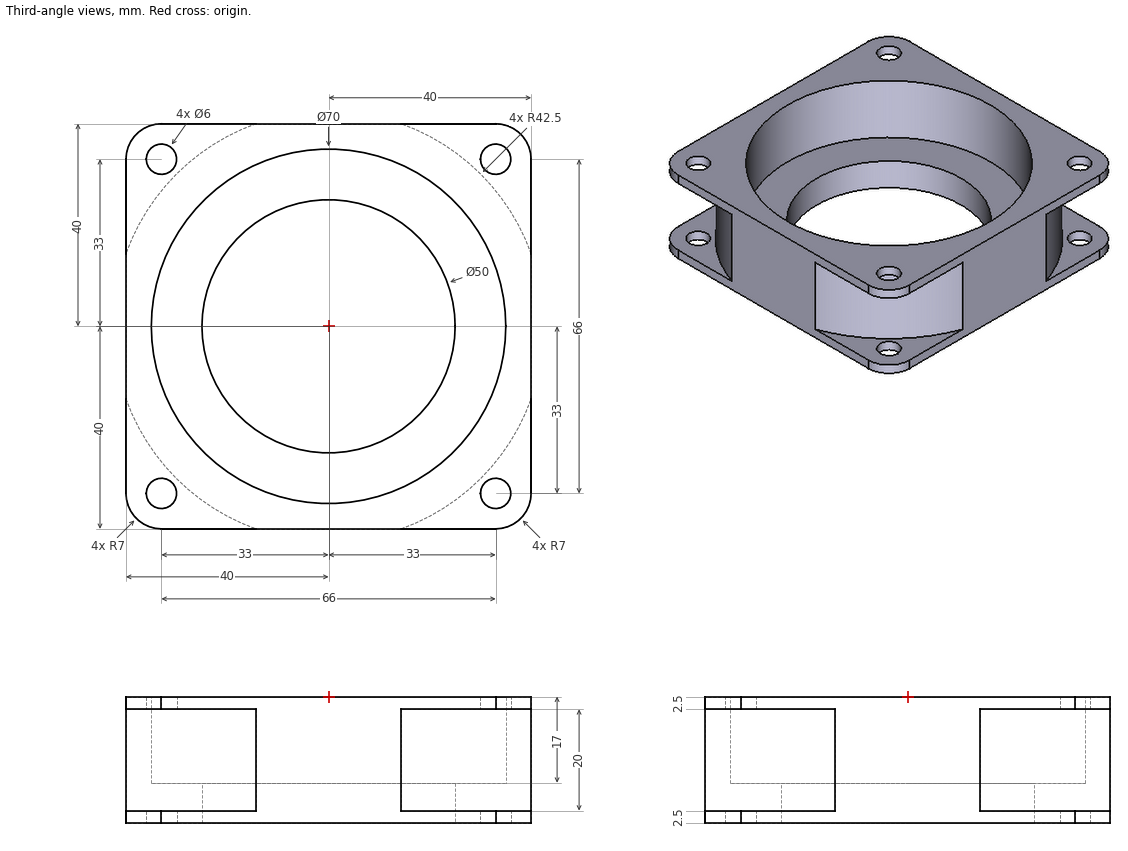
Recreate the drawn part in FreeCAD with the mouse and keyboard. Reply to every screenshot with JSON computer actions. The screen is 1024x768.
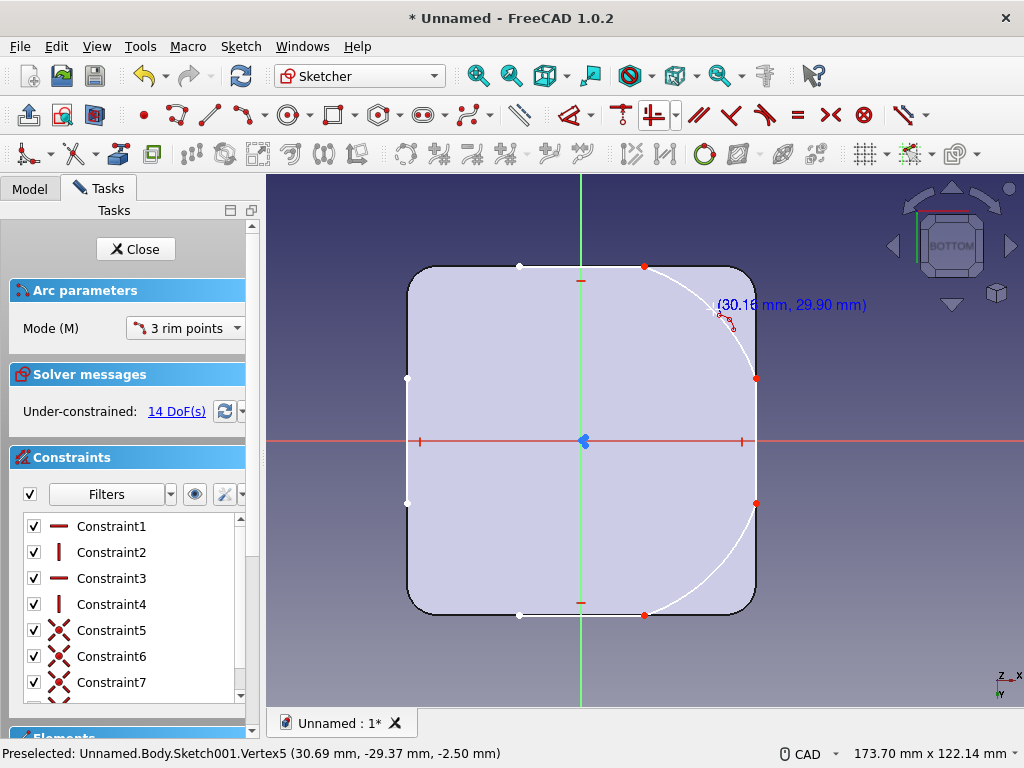
{"action": "left_click", "coordinate": [519, 267]}
{"action": "left_click", "coordinate": [407, 379]}
{"action": "left_click", "coordinate": [450, 309]}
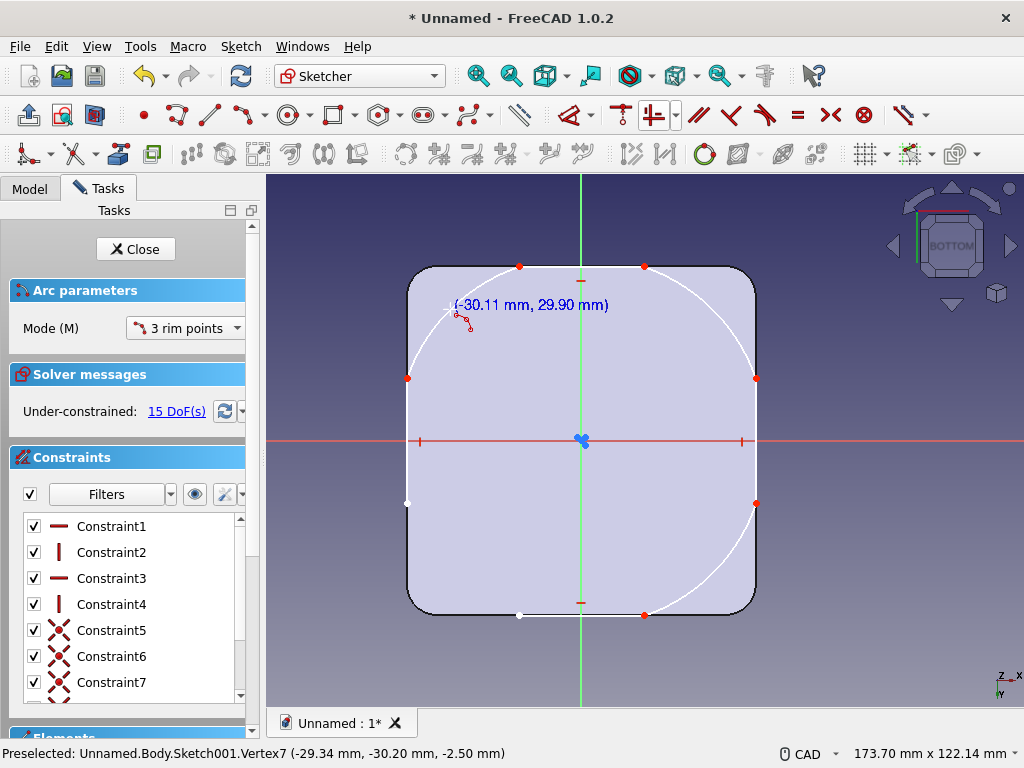
{"action": "left_click", "coordinate": [407, 504]}
{"action": "left_click", "coordinate": [519, 616]}
{"action": "left_click", "coordinate": [450, 572]}
{"action": "key", "text": "Escape"}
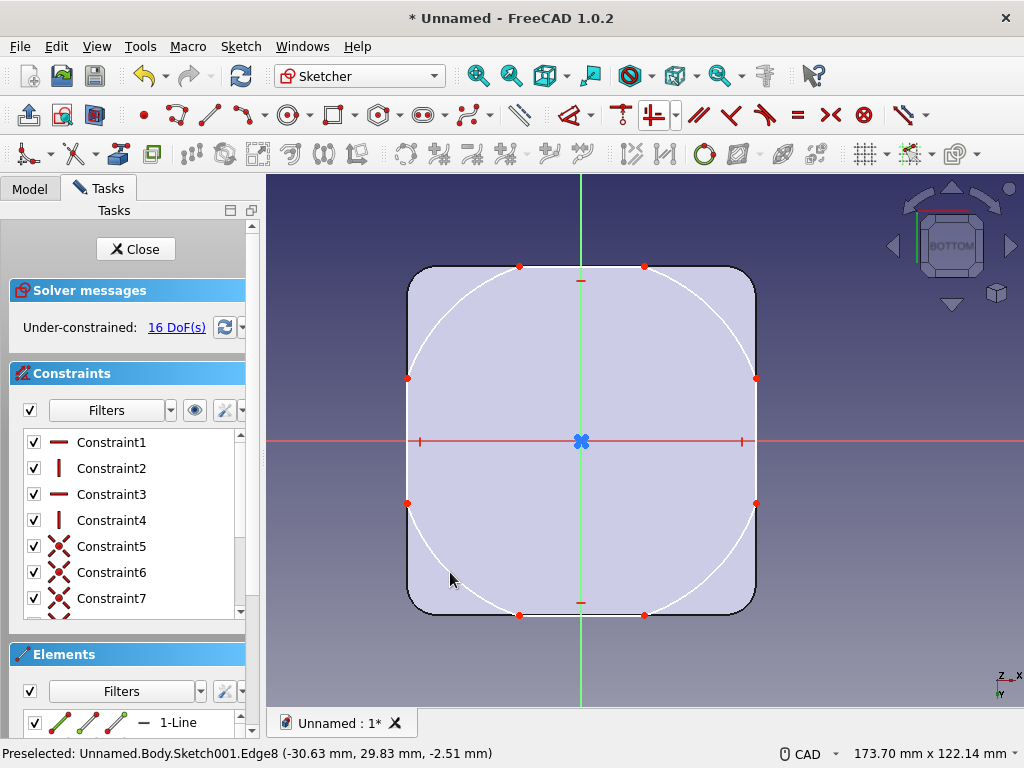
{"action": "left_click", "coordinate": [688, 594]}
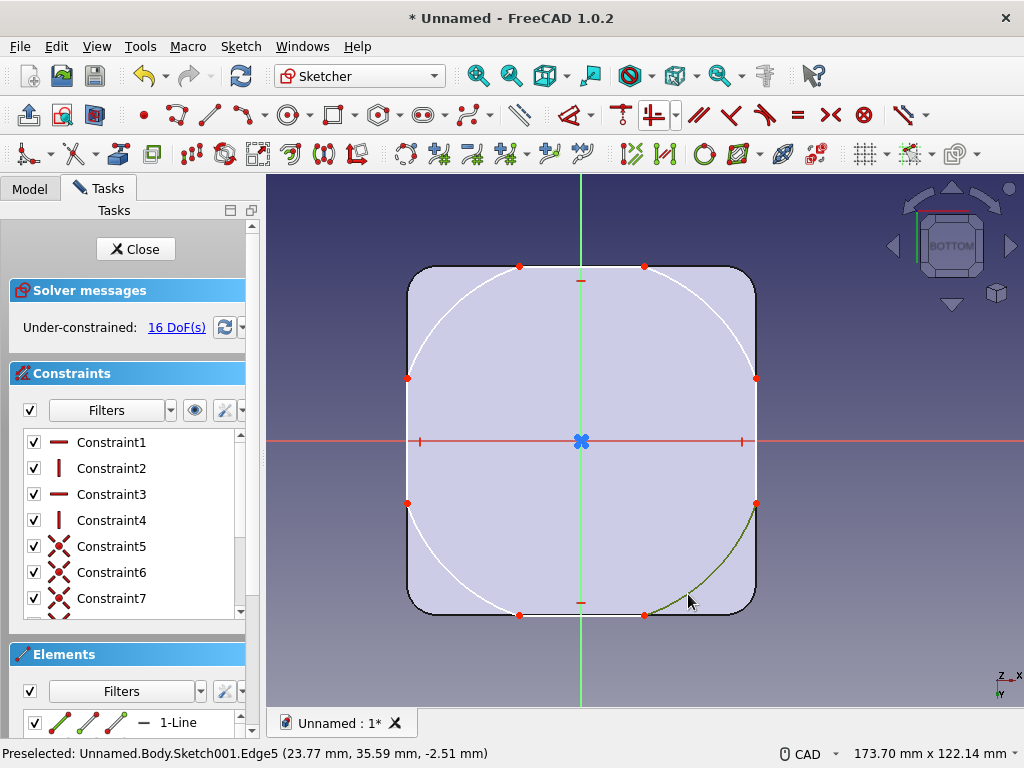
{"action": "left_click", "coordinate": [734, 335]}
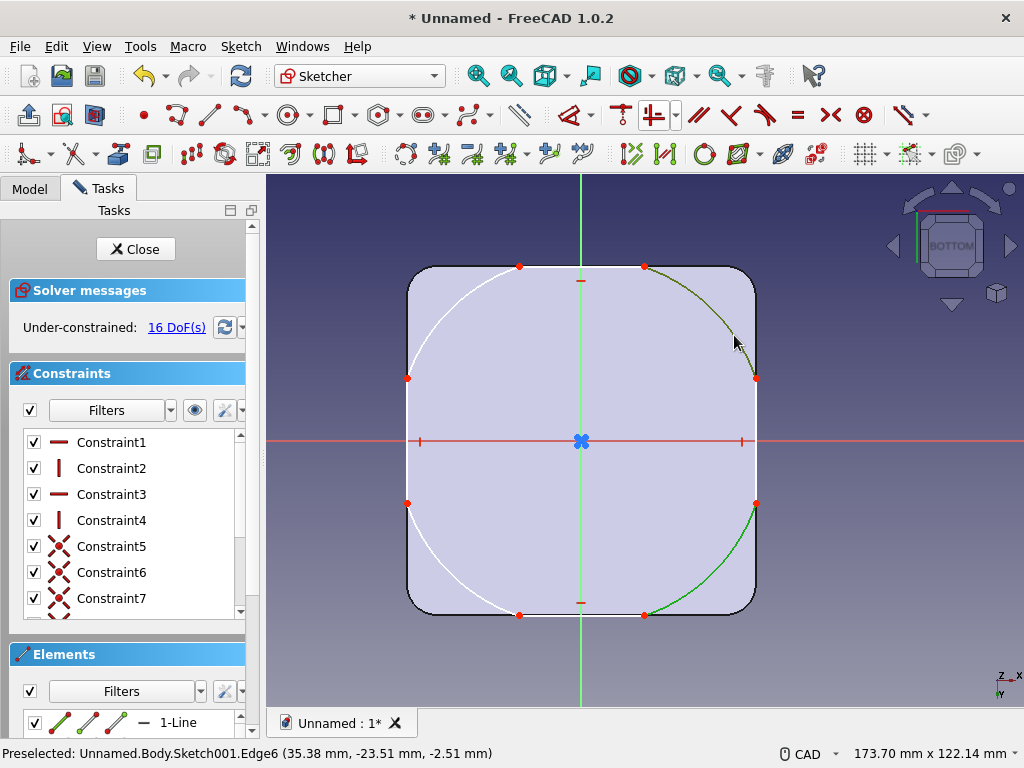
{"action": "left_click", "coordinate": [621, 116]}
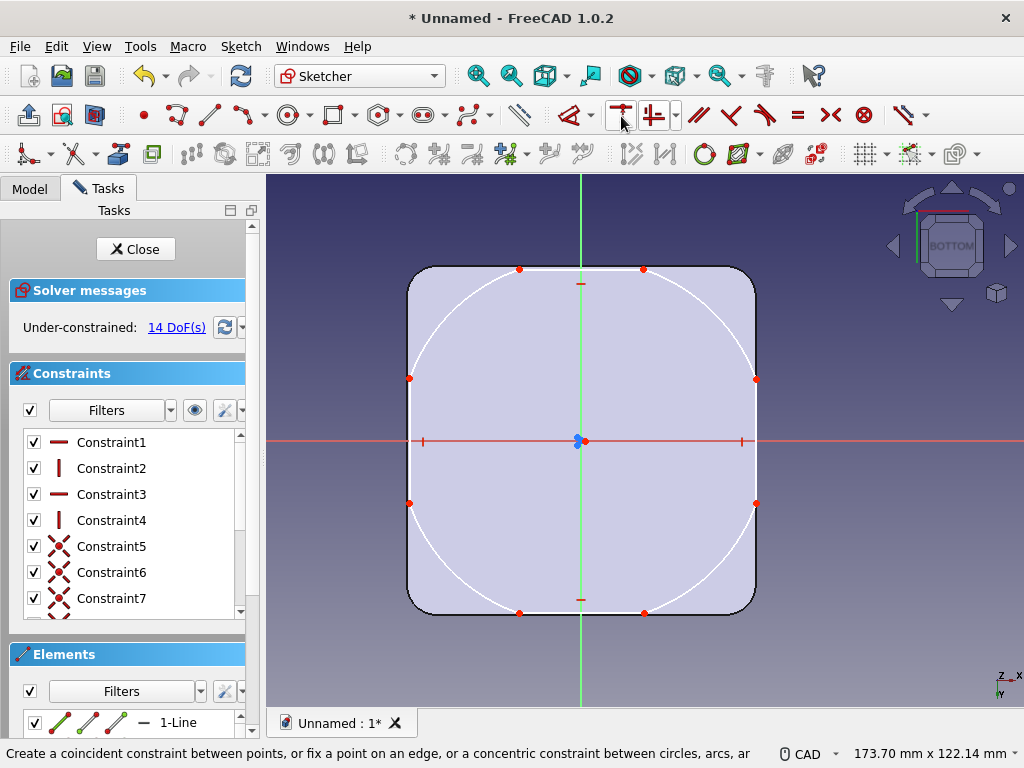
{"action": "left_click", "coordinate": [687, 592]}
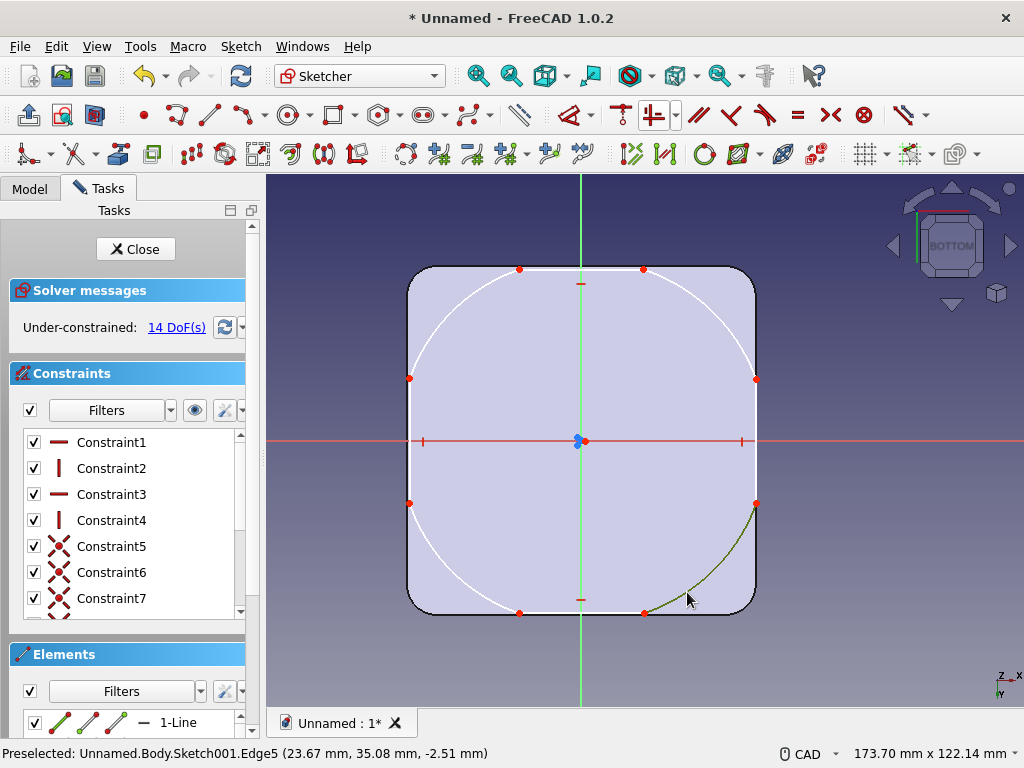
{"action": "left_click", "coordinate": [476, 291]}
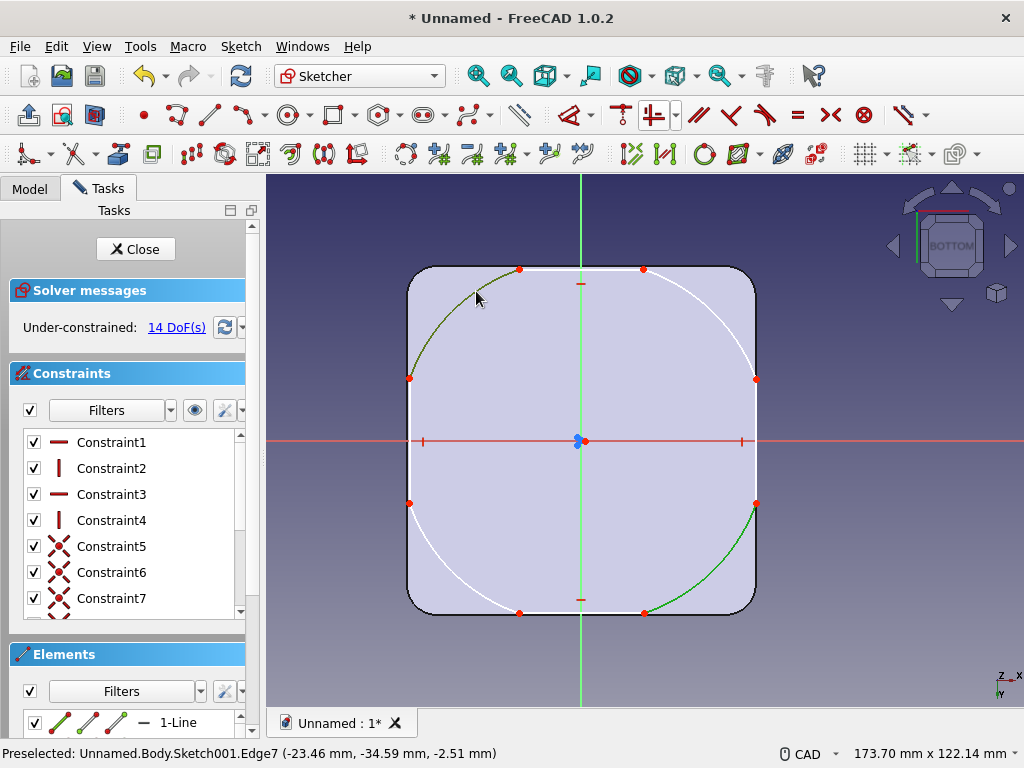
{"action": "left_click", "coordinate": [621, 116]}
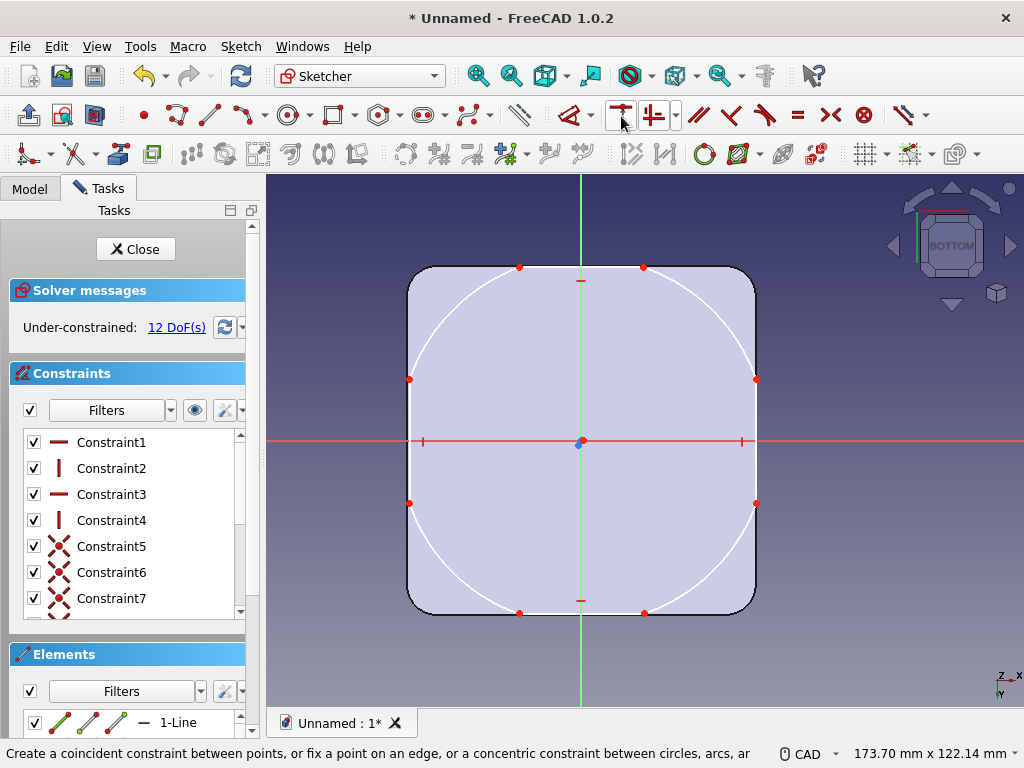
{"action": "left_click", "coordinate": [687, 592]}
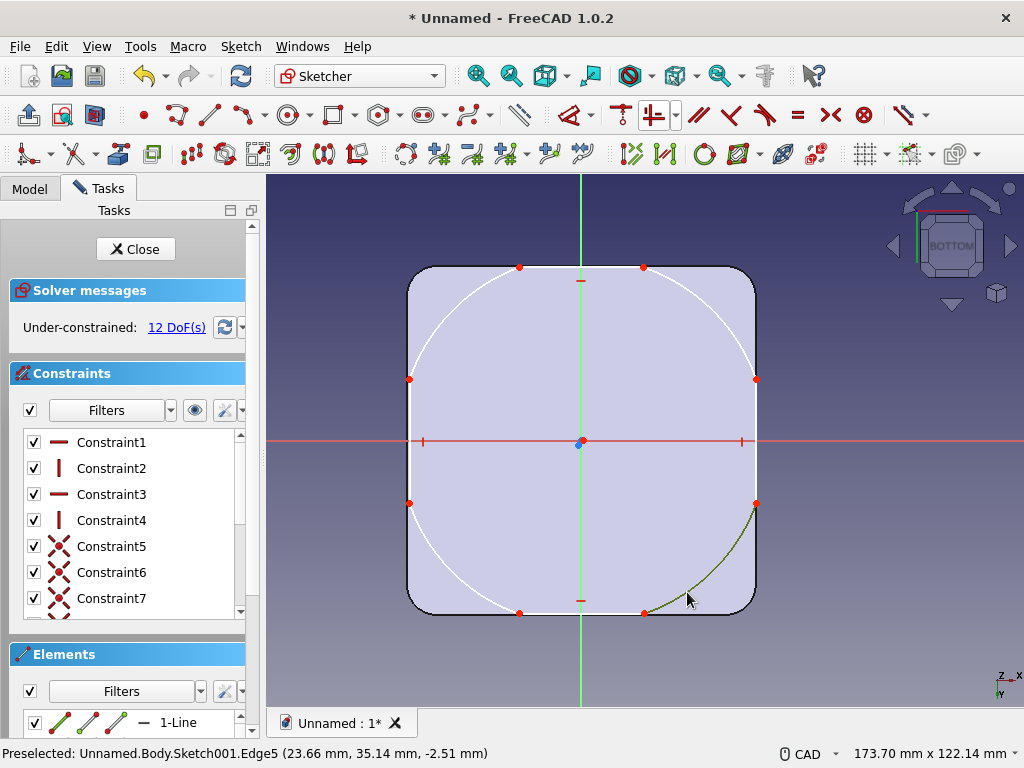
{"action": "left_click", "coordinate": [431, 547]}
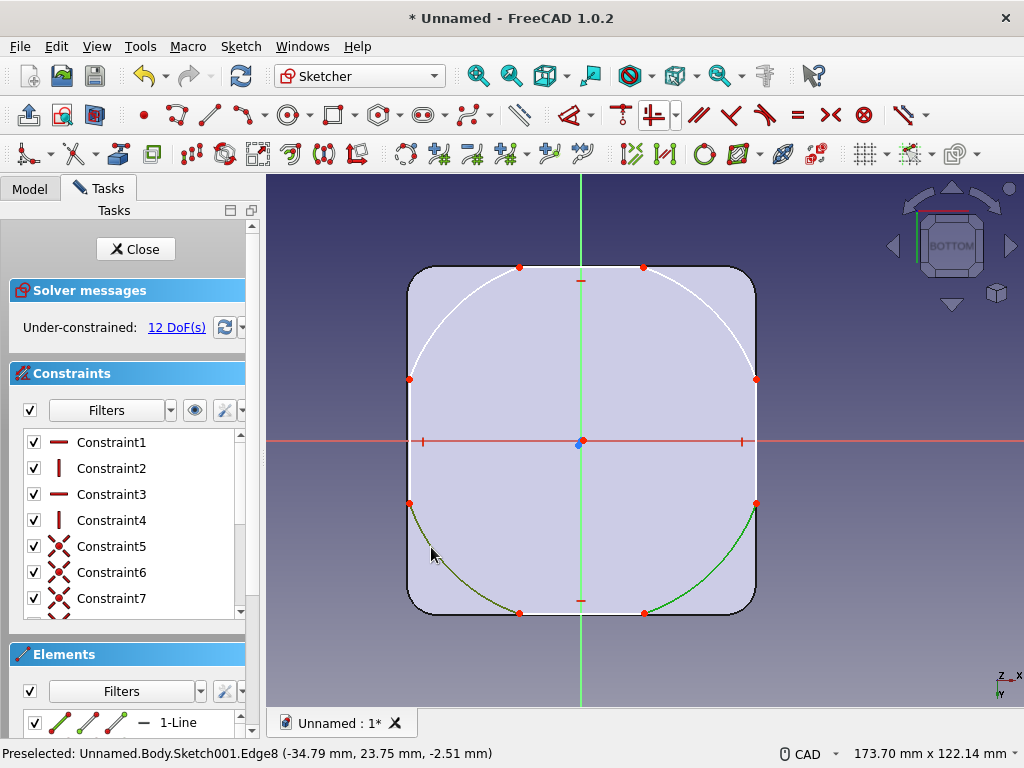
{"action": "left_click", "coordinate": [621, 116]}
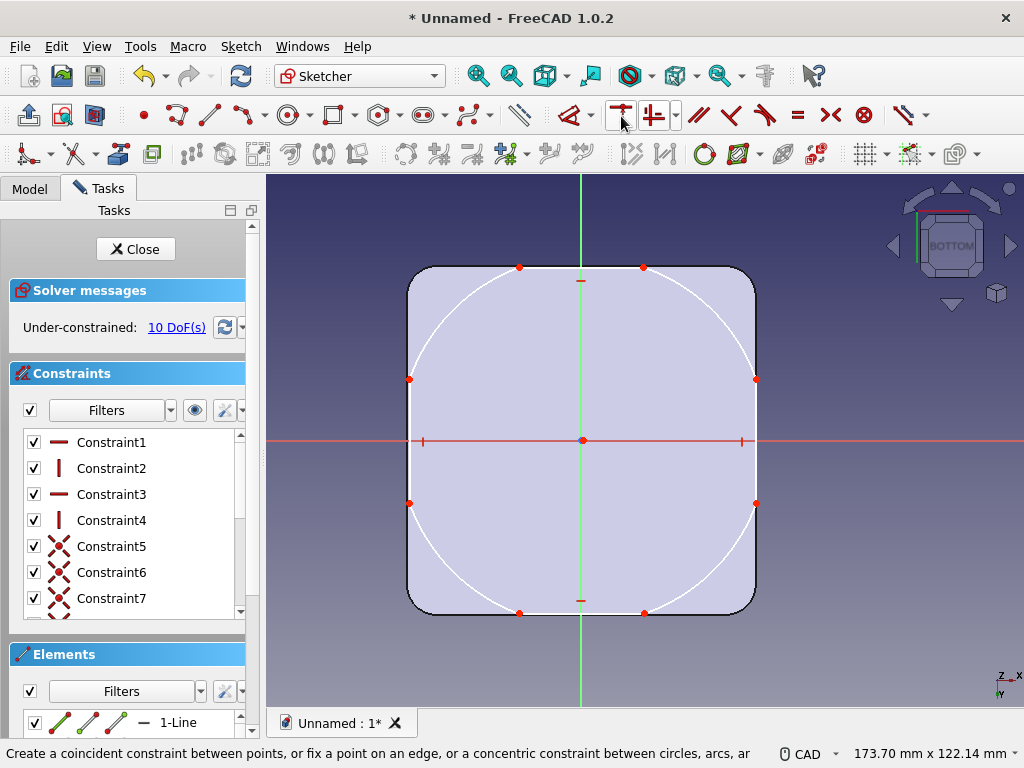
{"action": "left_click_drag", "start_coordinate": [571, 430], "coordinate": [594, 450]}